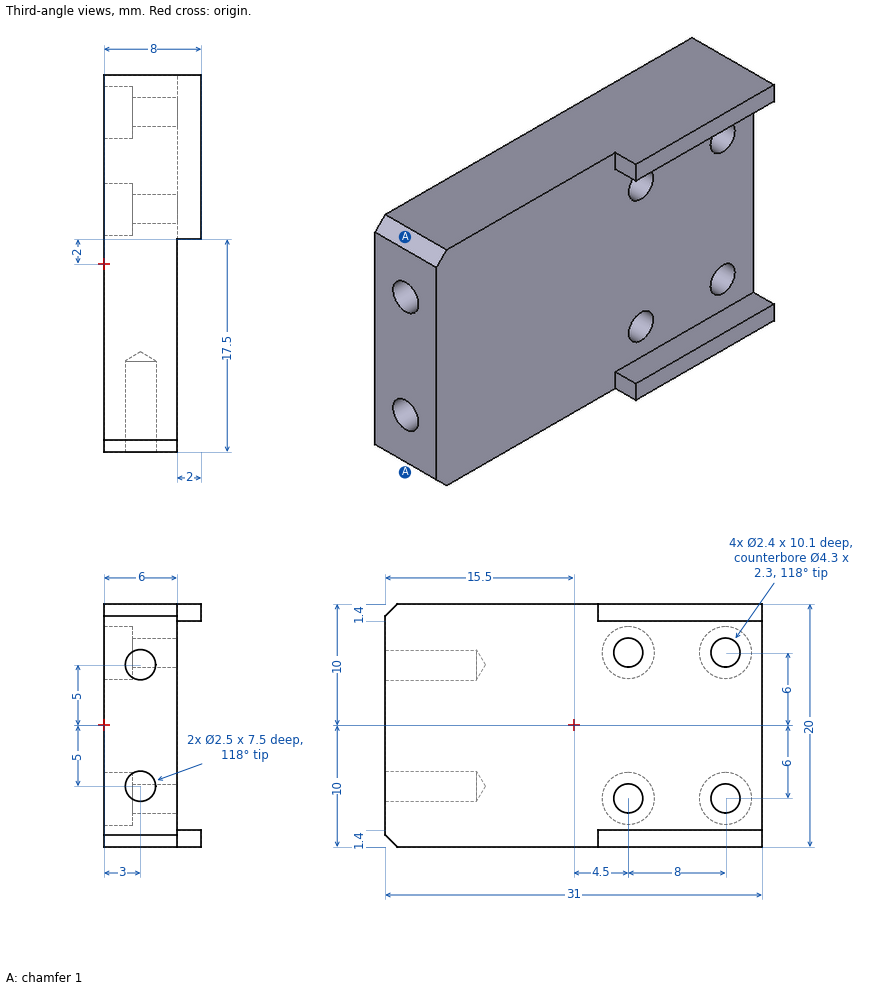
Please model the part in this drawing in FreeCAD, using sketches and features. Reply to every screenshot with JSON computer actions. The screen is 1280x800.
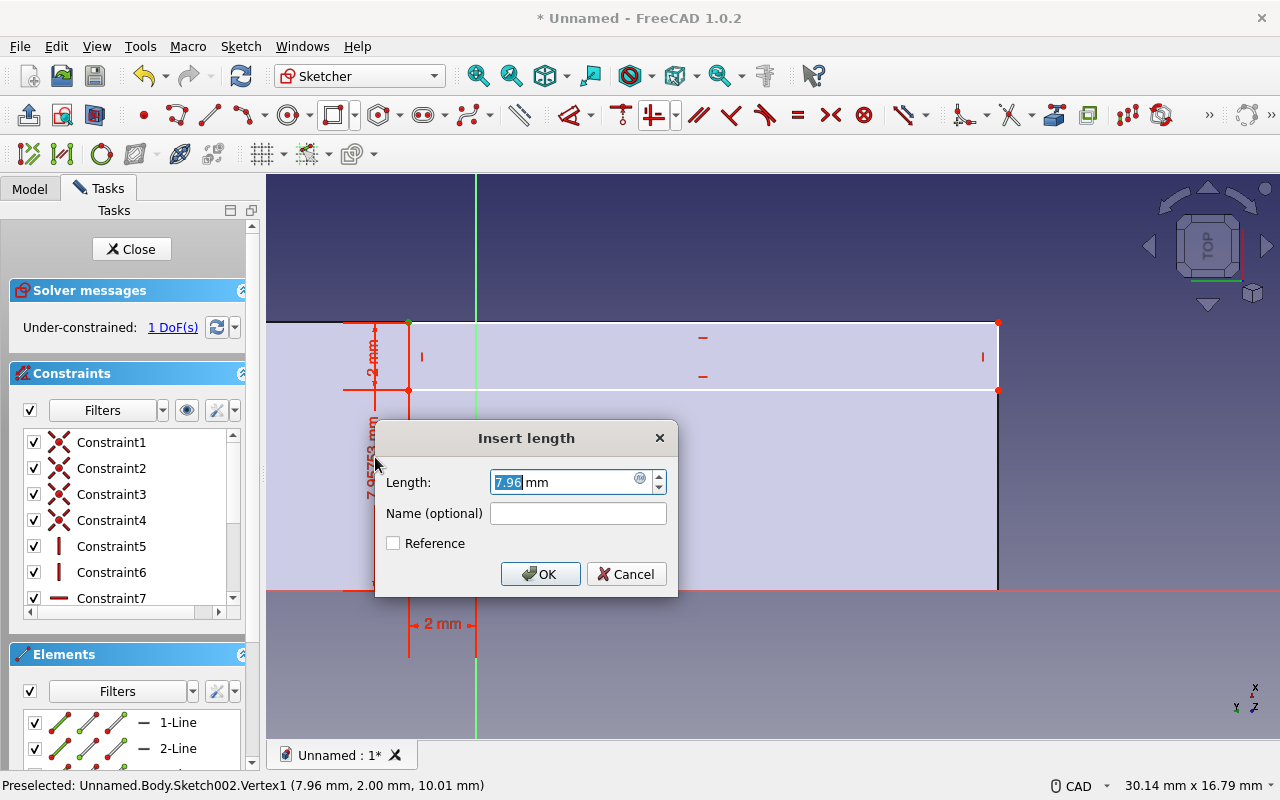
{"action": "type", "text": "8"}
{"action": "key", "text": "Return"}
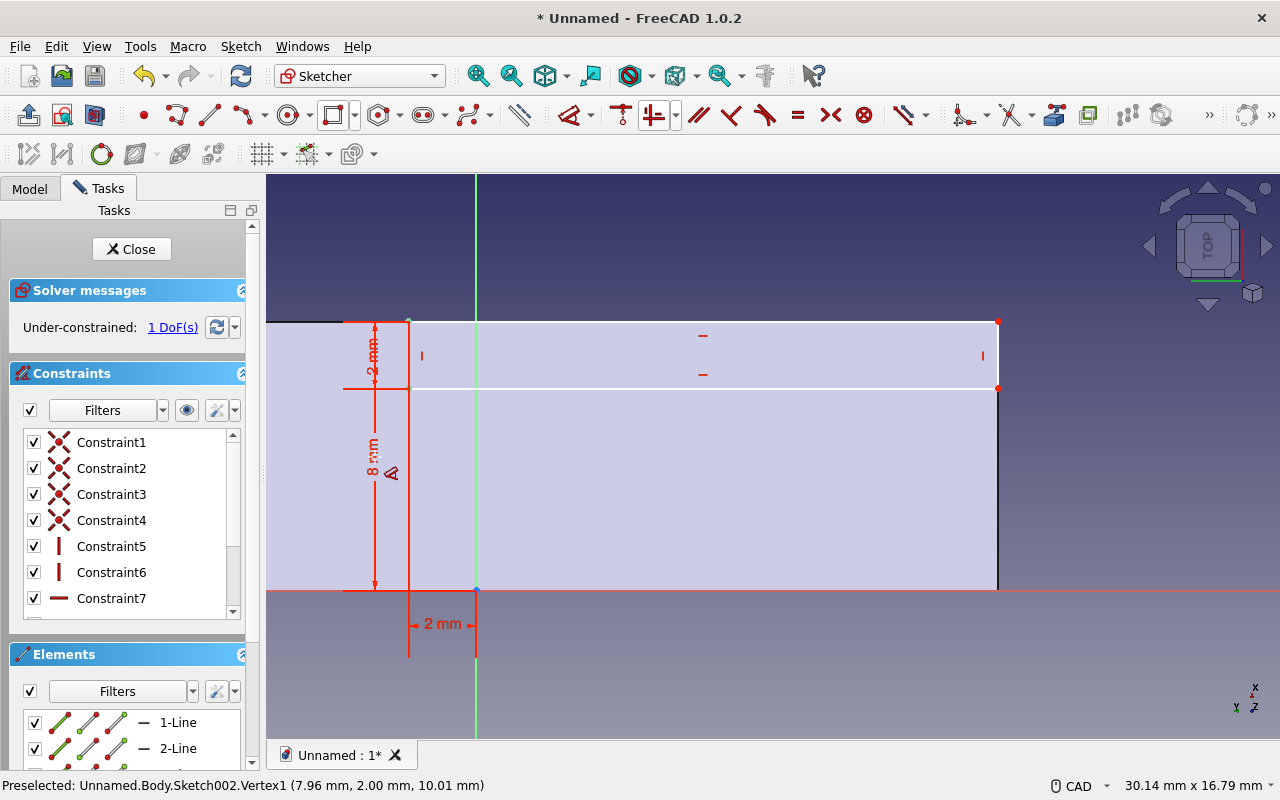
{"action": "left_click", "coordinate": [586, 389]}
{"action": "left_click", "coordinate": [703, 355]}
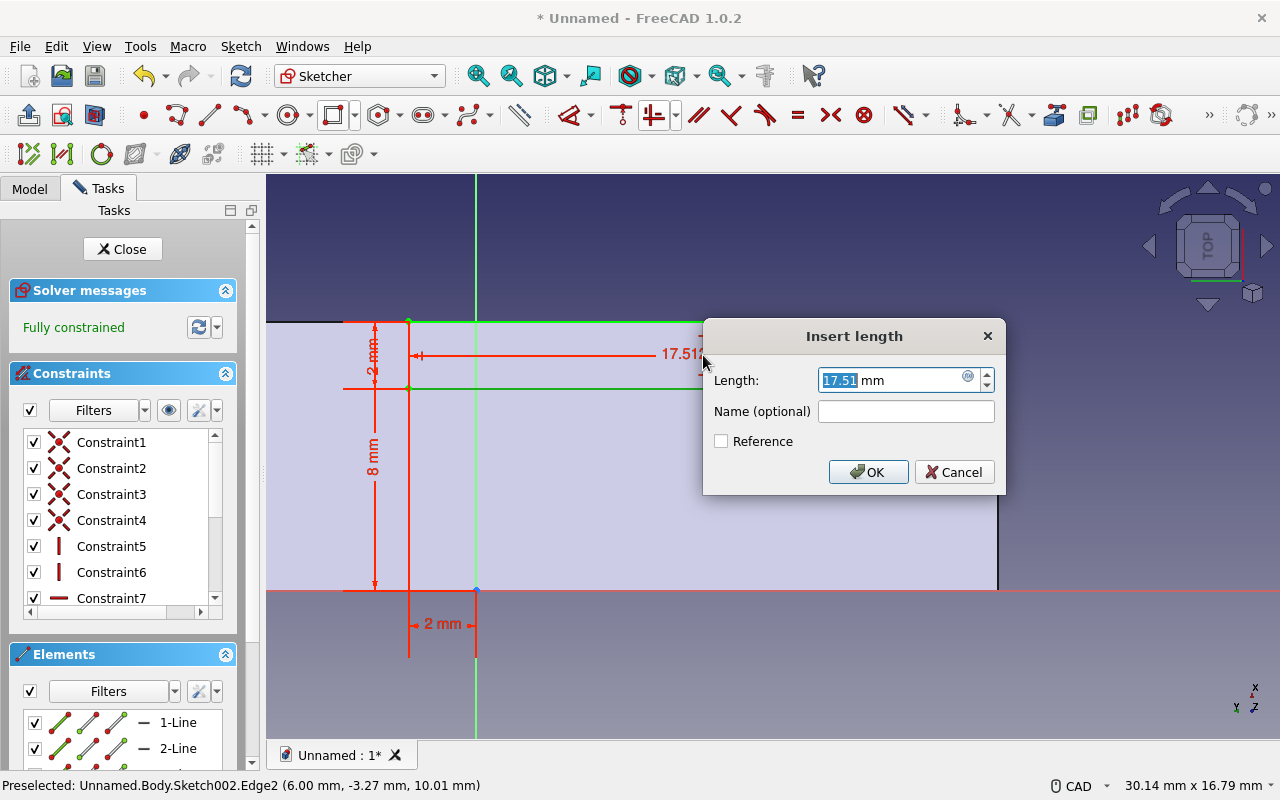
{"action": "type", "text": "17.5"}
{"action": "key", "text": "Return"}
{"action": "key", "text": "Escape"}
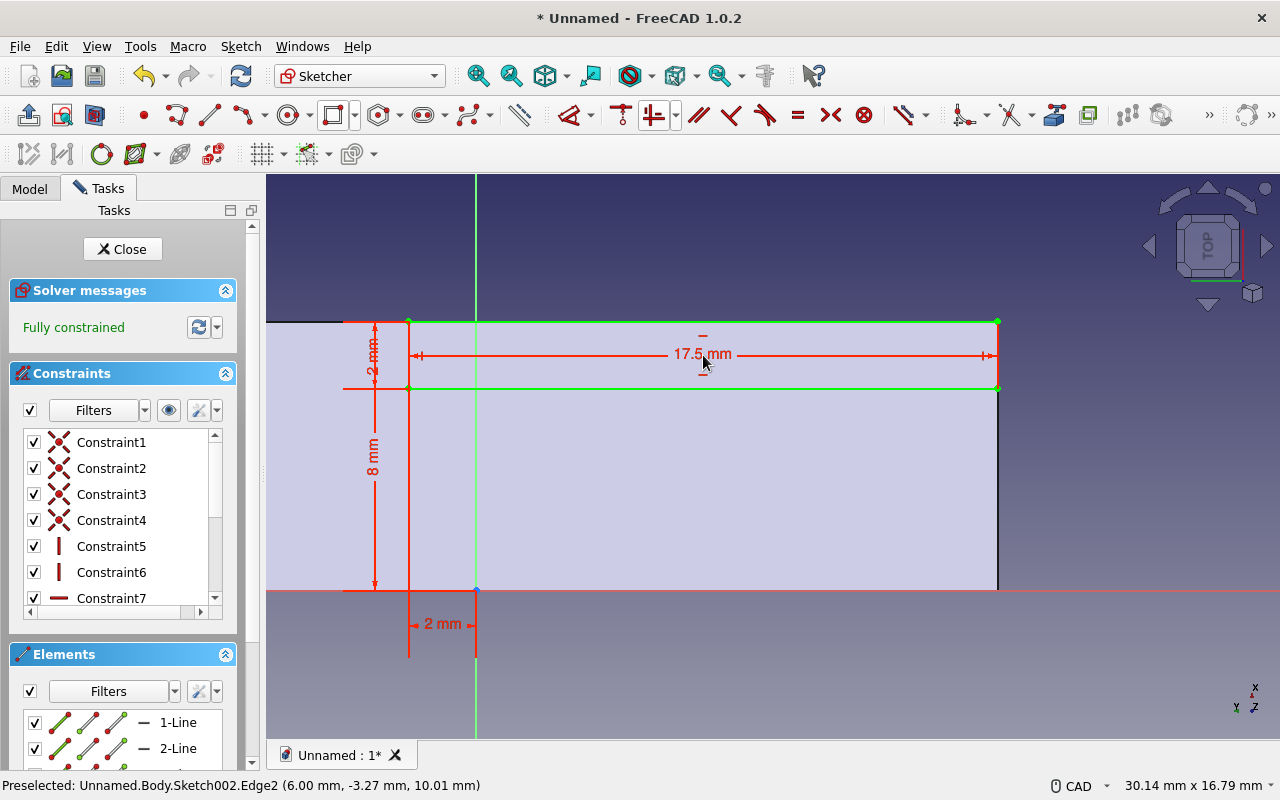
{"action": "left_click", "coordinate": [123, 249]}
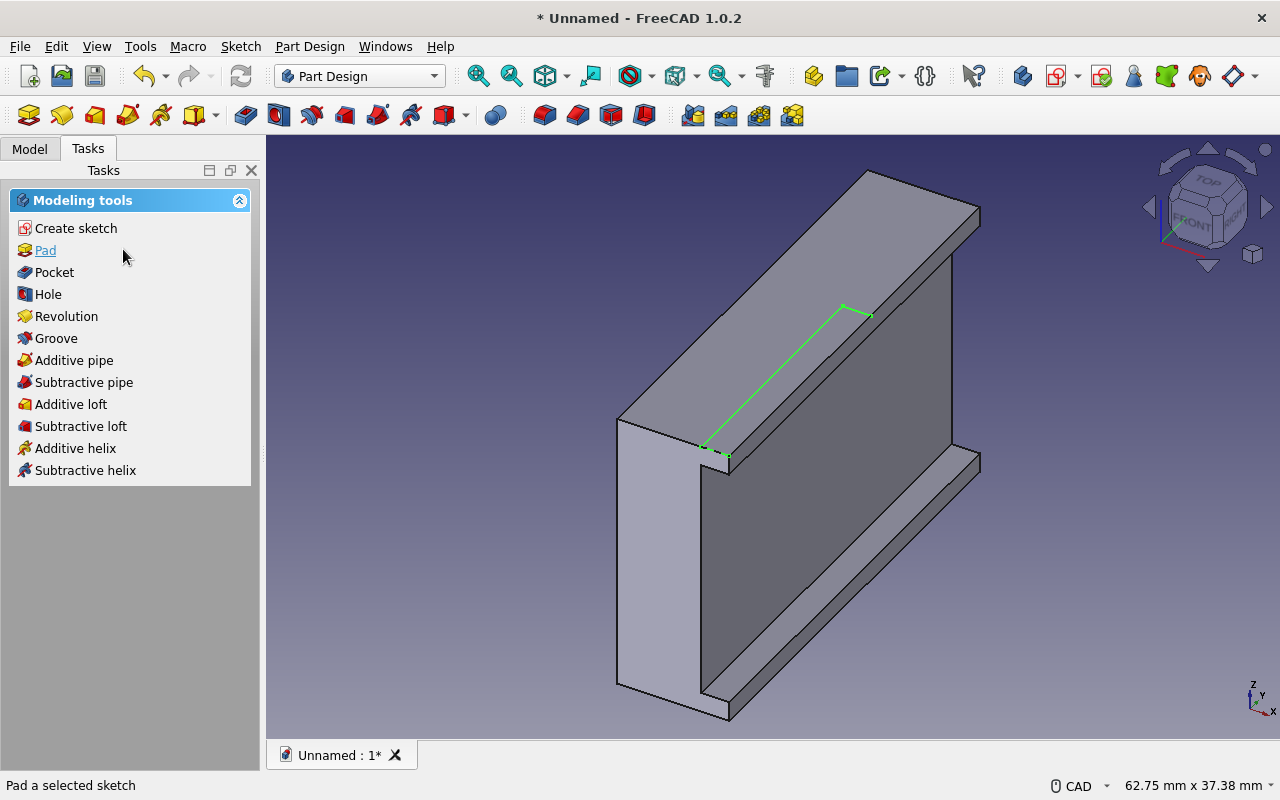
{"action": "left_click", "coordinate": [246, 116]}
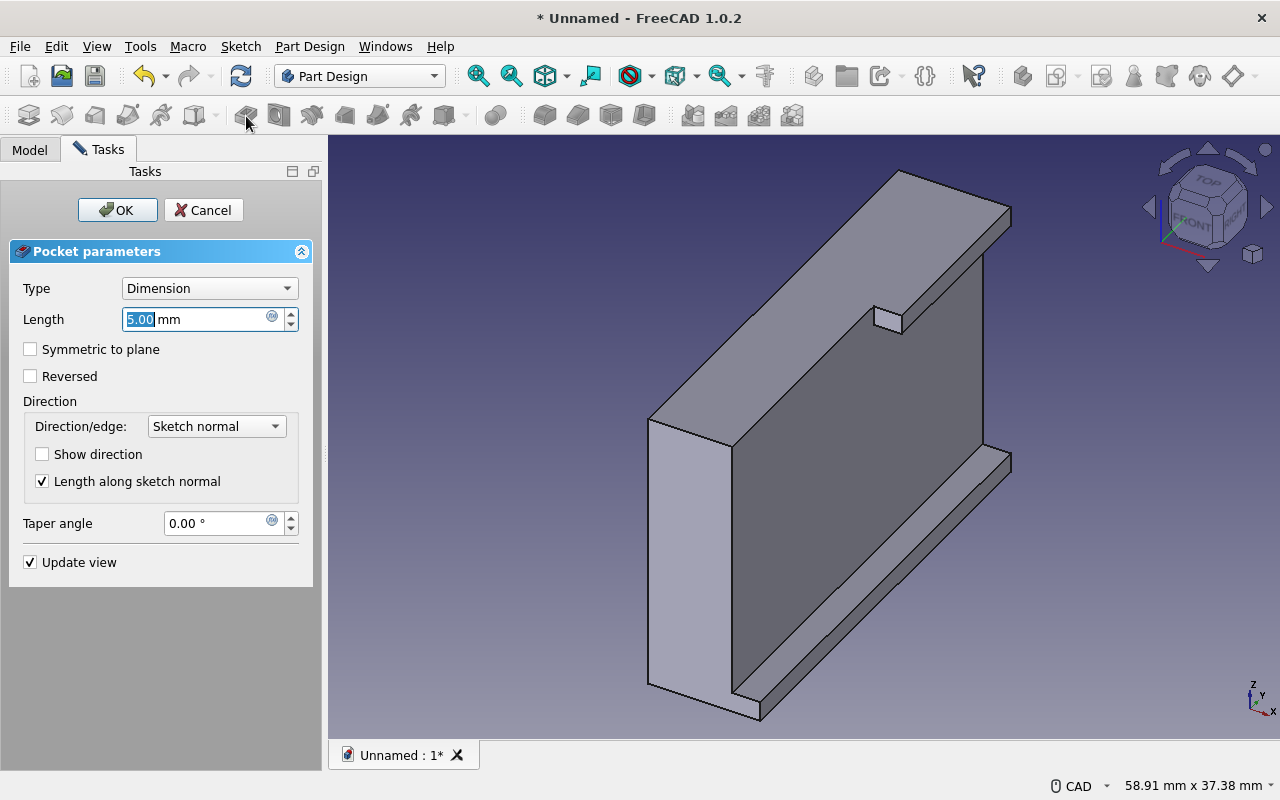
{"action": "left_click", "coordinate": [210, 288]}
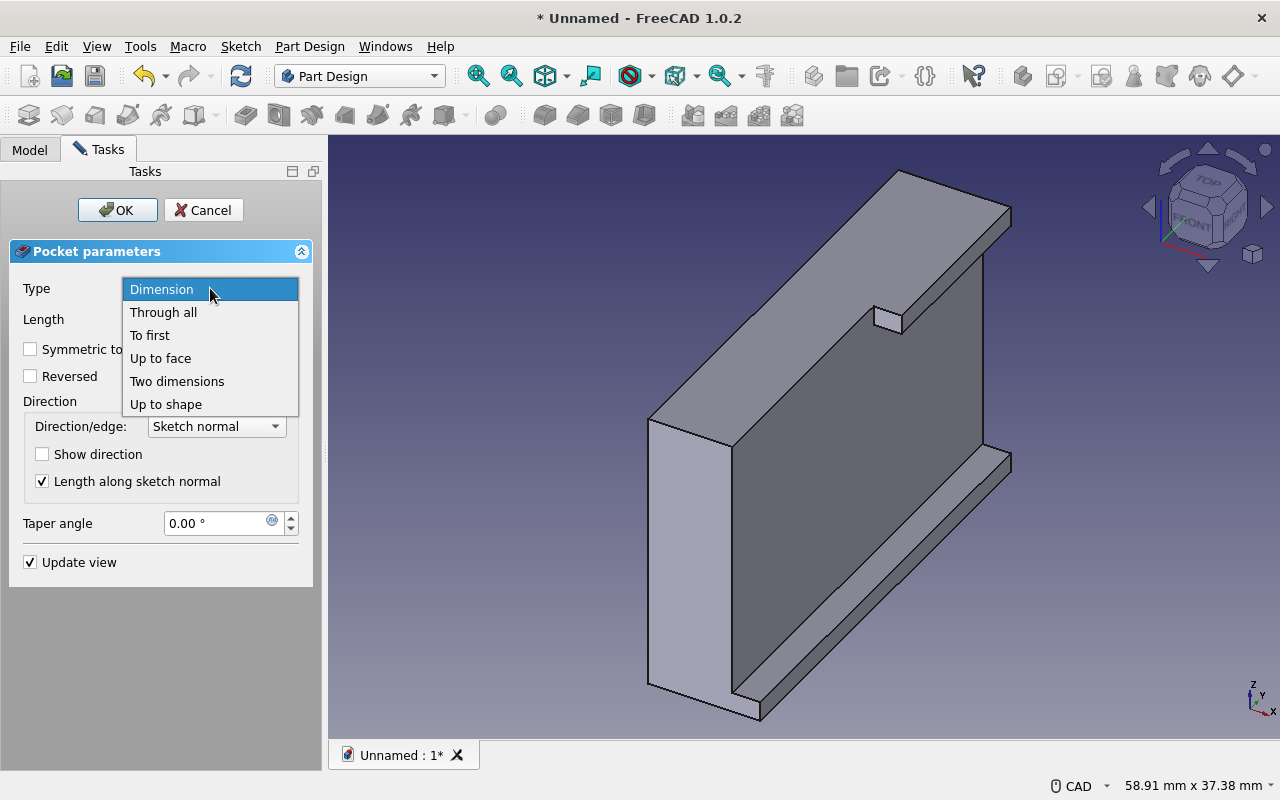
{"action": "left_click", "coordinate": [208, 312]}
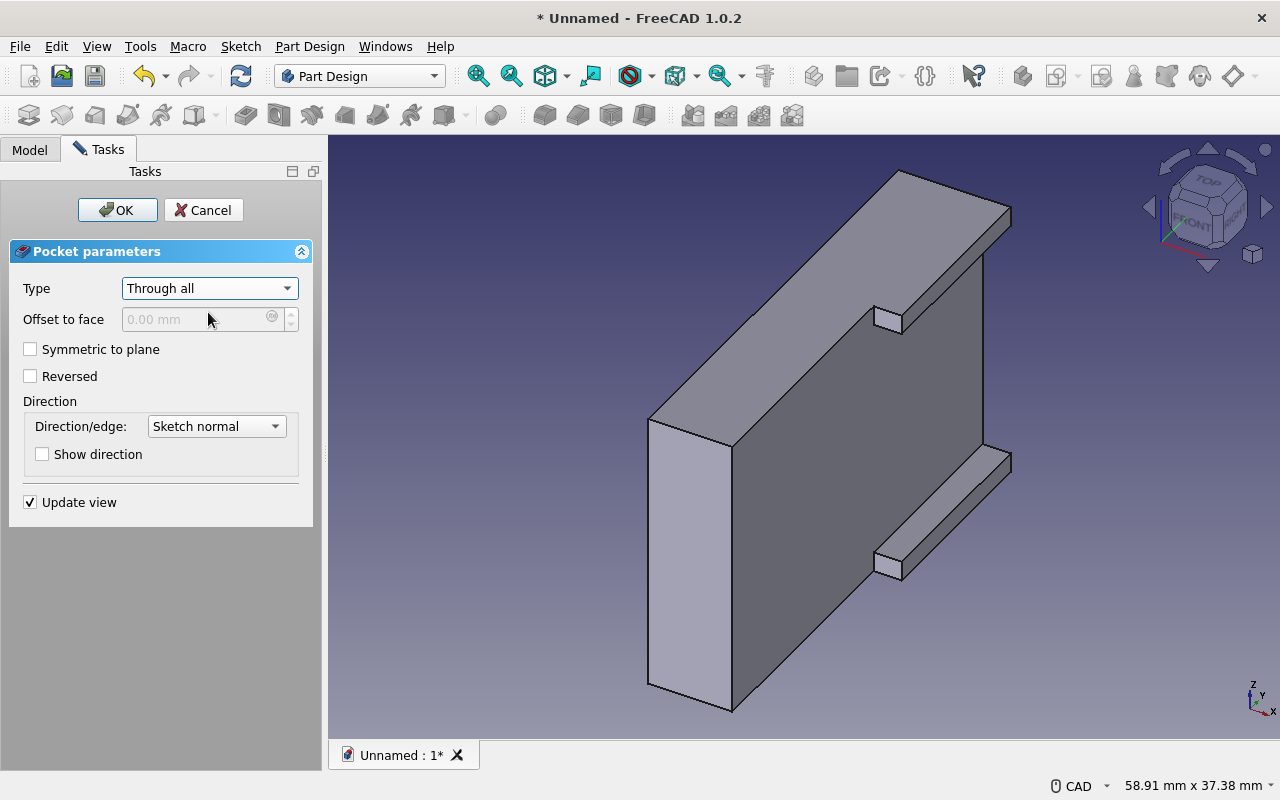
{"action": "left_click", "coordinate": [118, 210]}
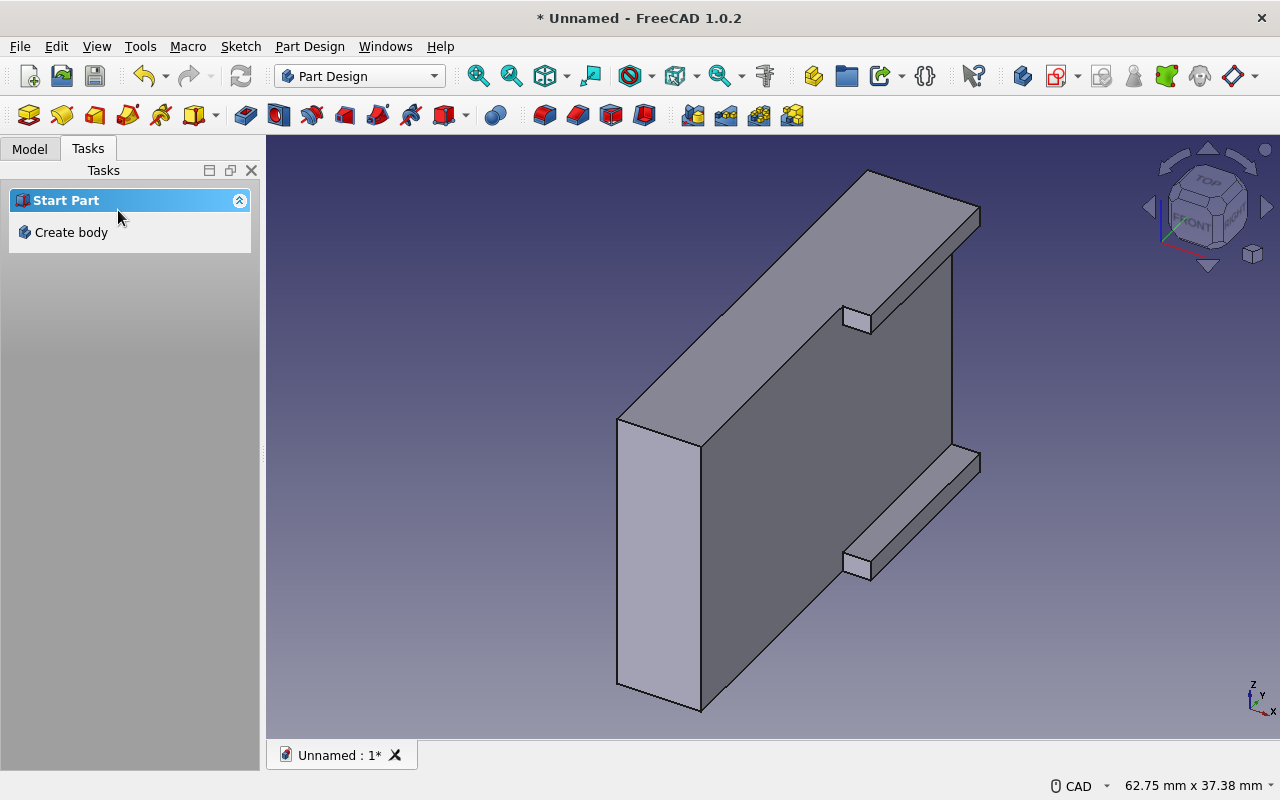
{"action": "left_click", "coordinate": [1056, 76]}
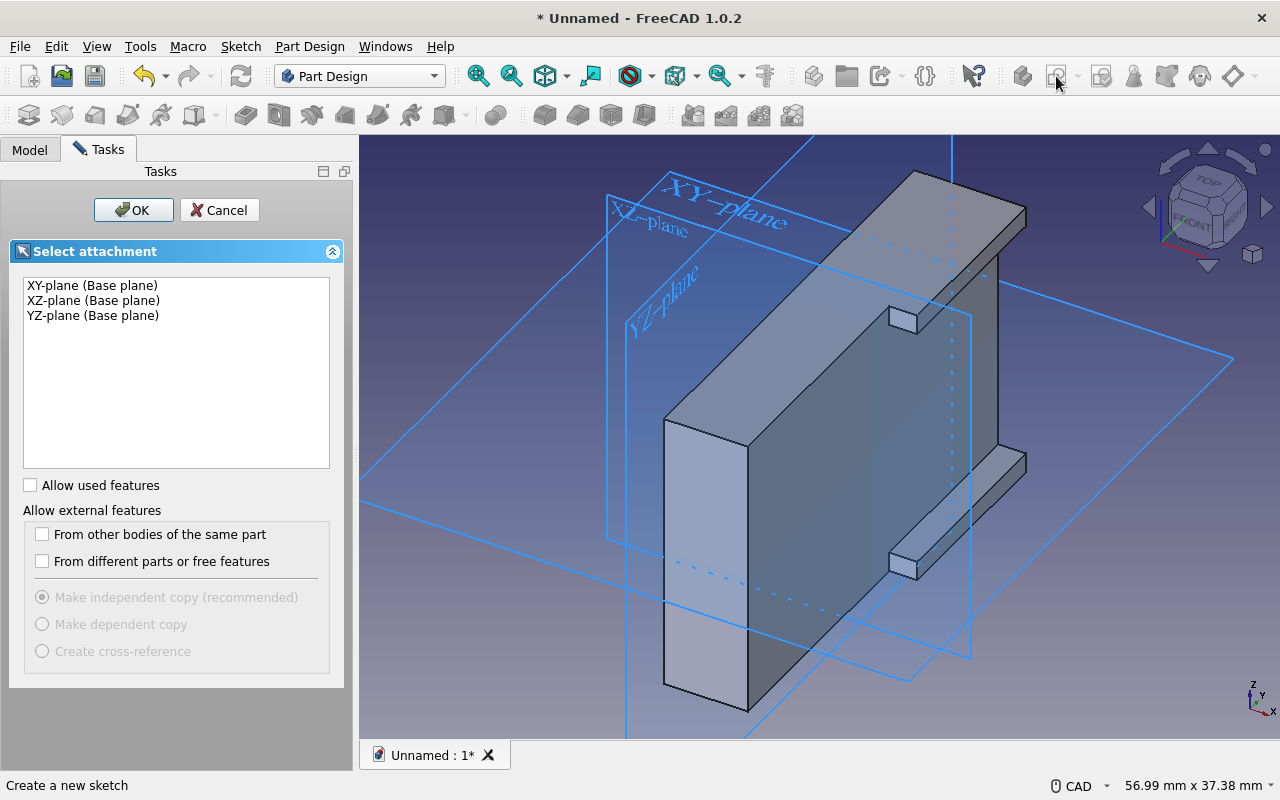
{"action": "left_click", "coordinate": [84, 316]}